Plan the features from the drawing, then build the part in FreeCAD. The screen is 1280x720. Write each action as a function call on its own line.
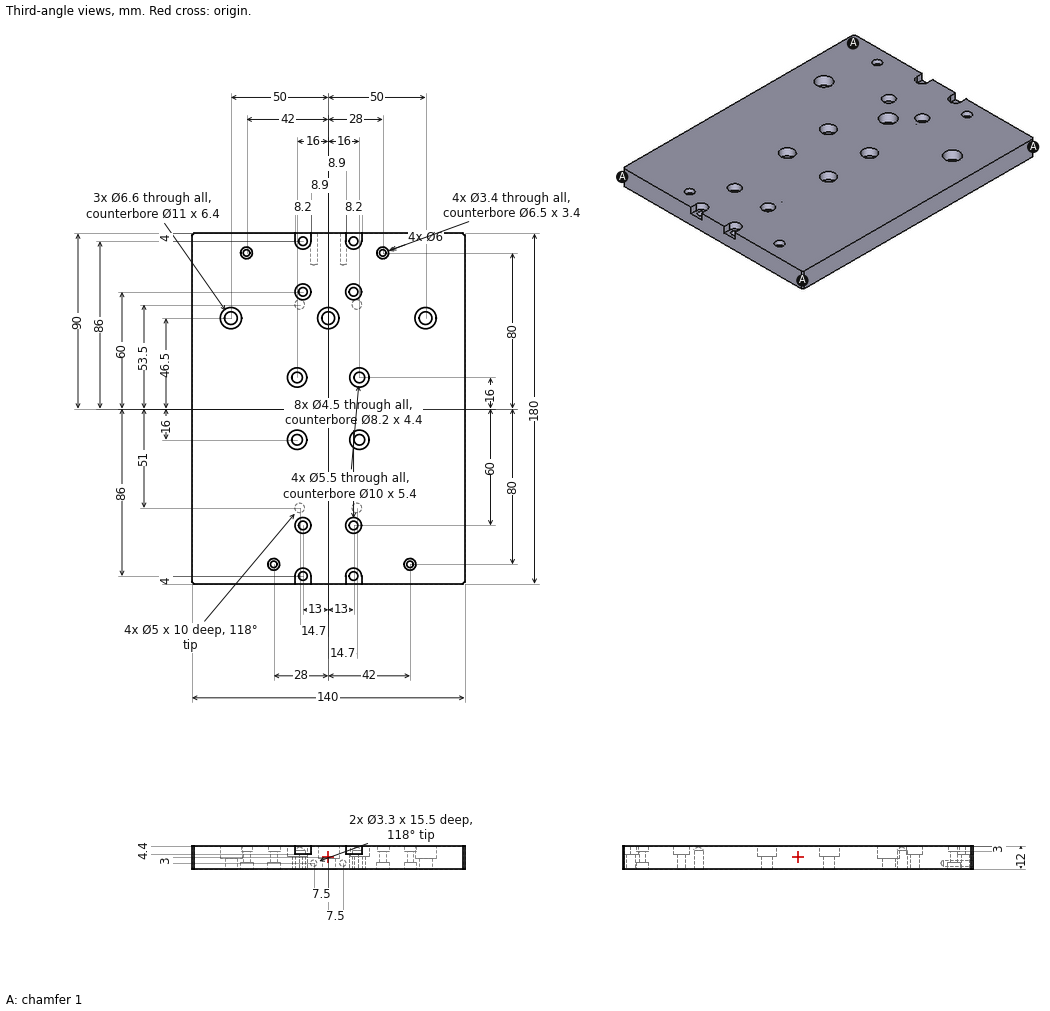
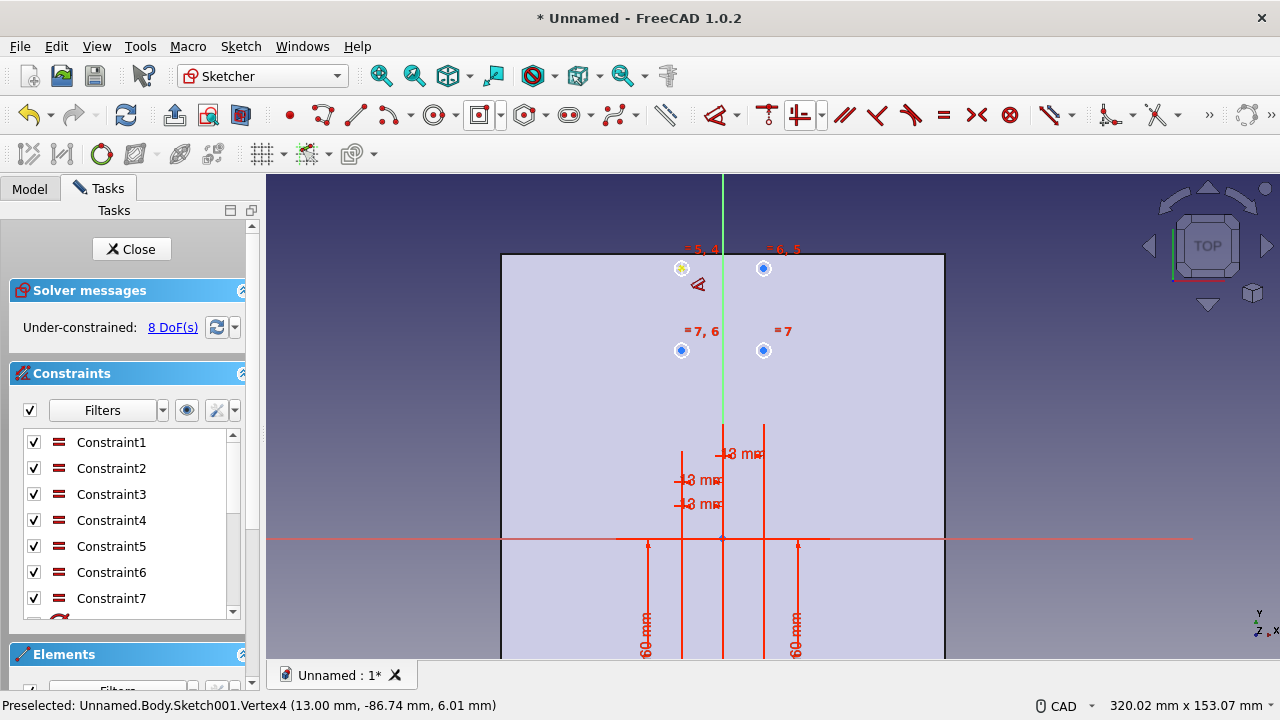
click(682, 269)
click(702, 235)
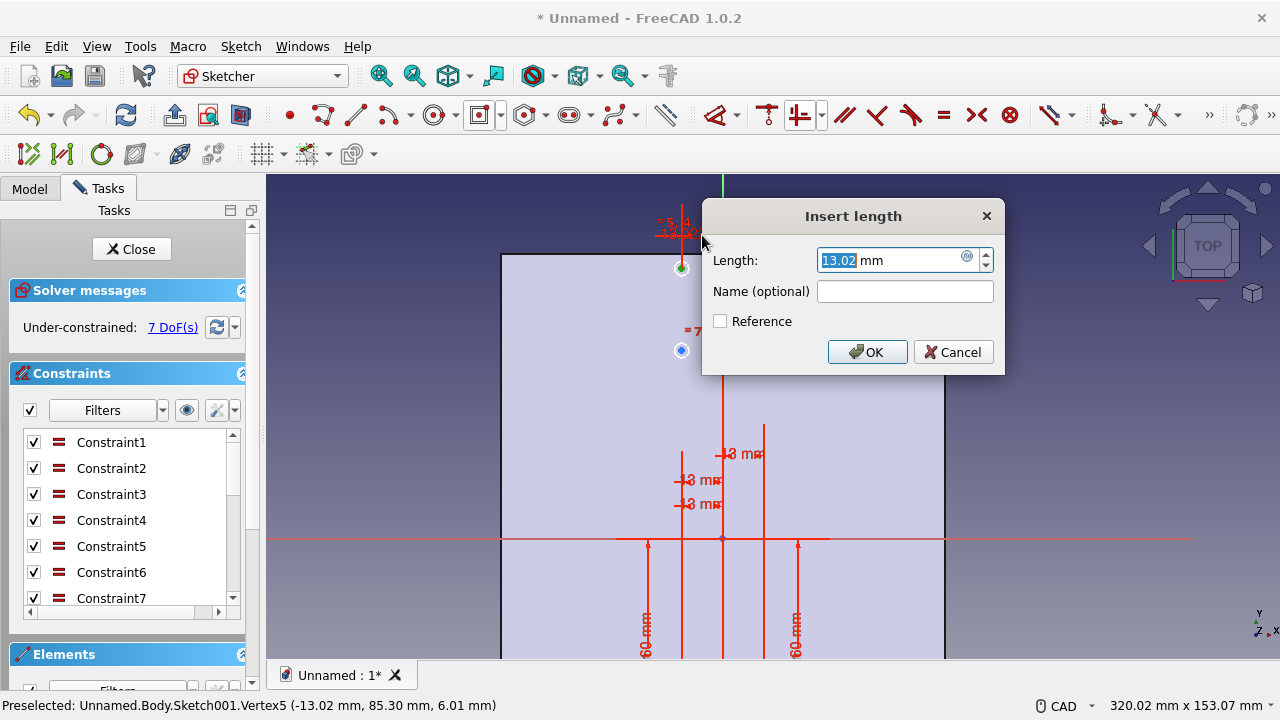
text(13)
key(Return)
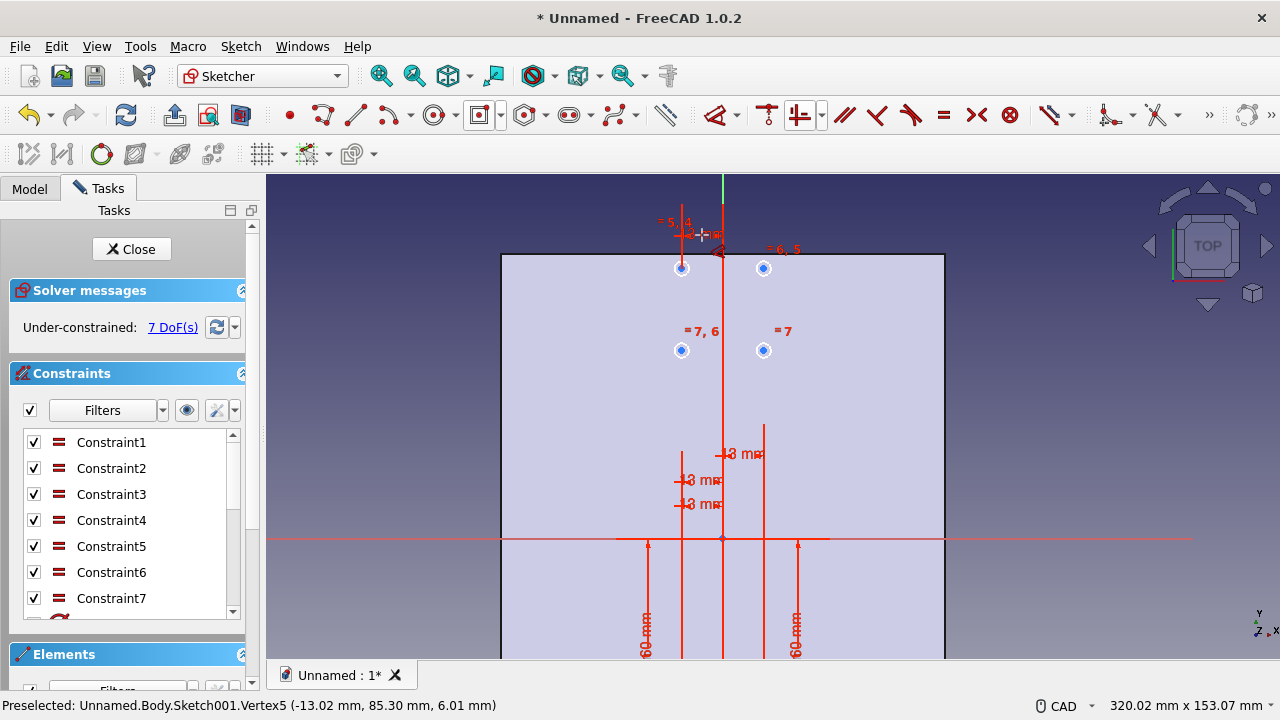
click(682, 269)
click(648, 404)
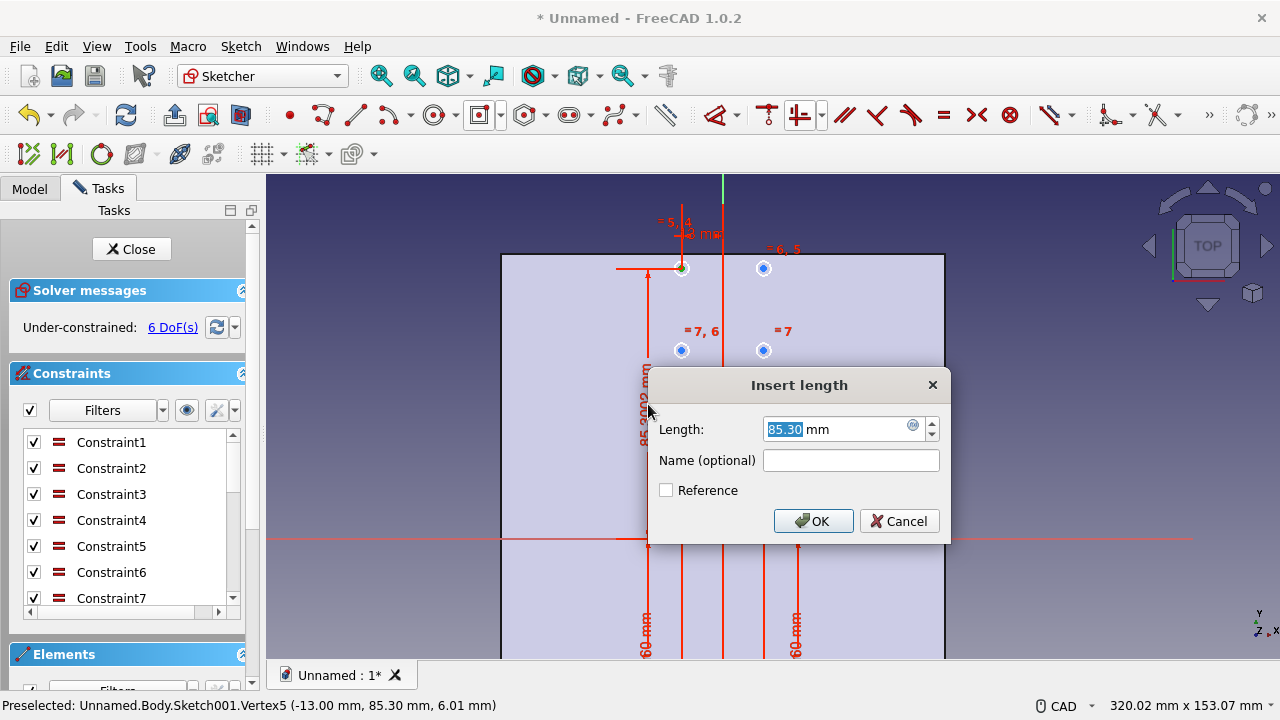
text(86)
key(Return)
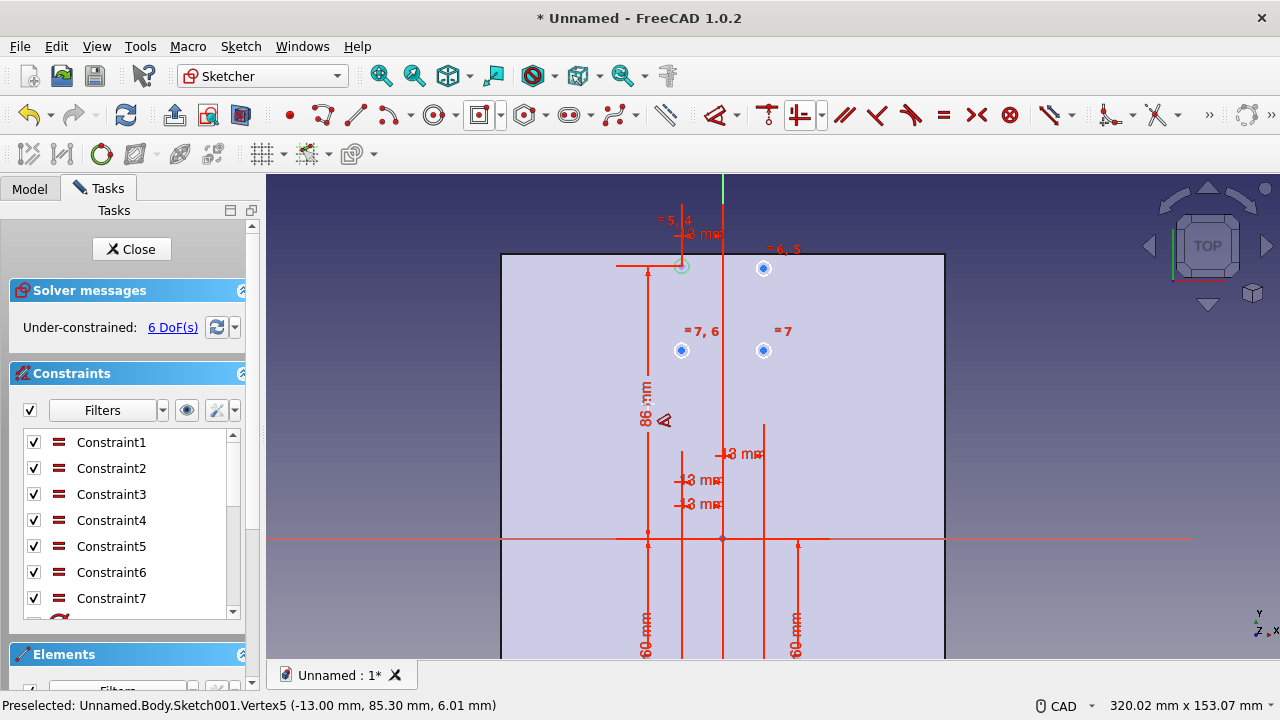
click(764, 269)
click(743, 573)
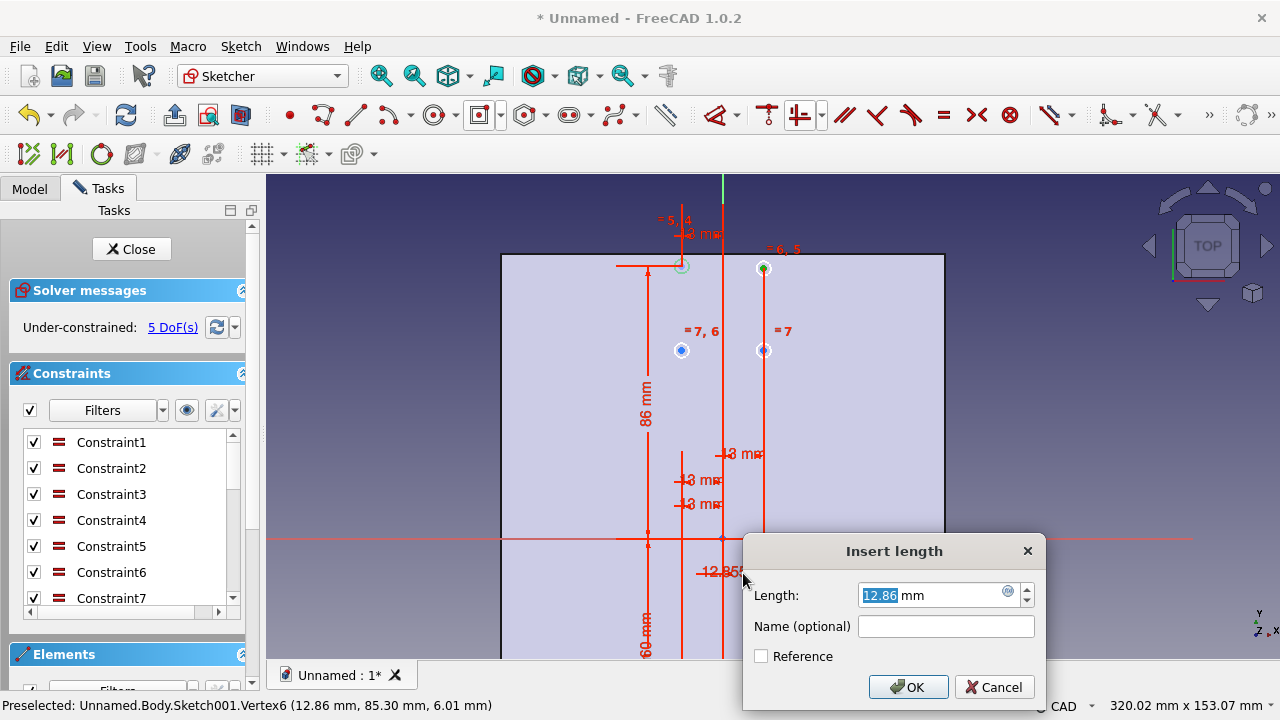
text(13)
key(Return)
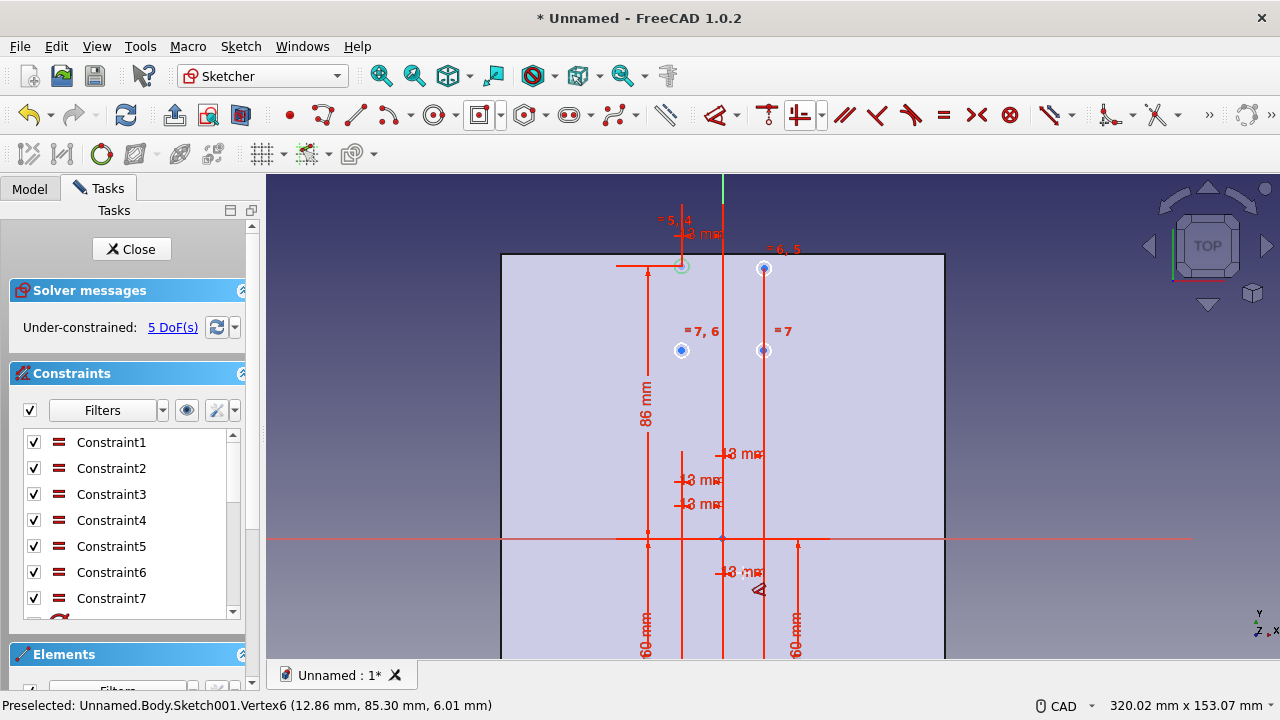
click(764, 269)
click(798, 404)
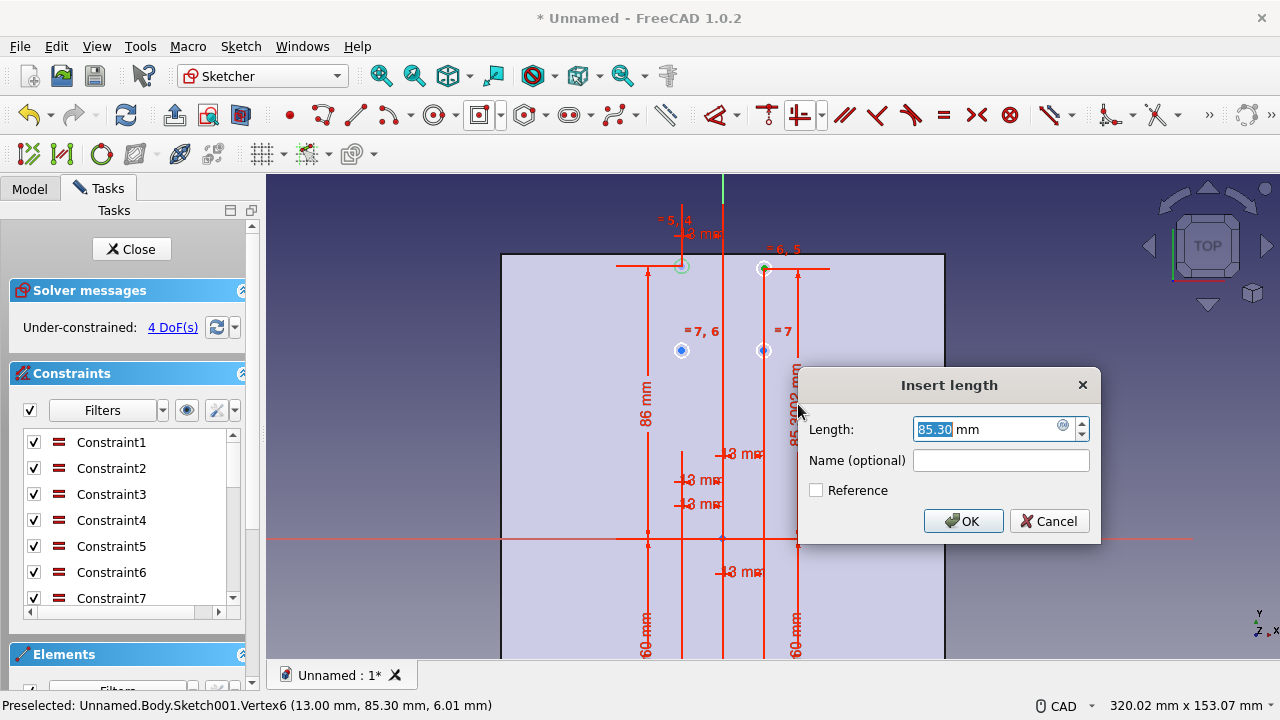
text(86)
key(Return)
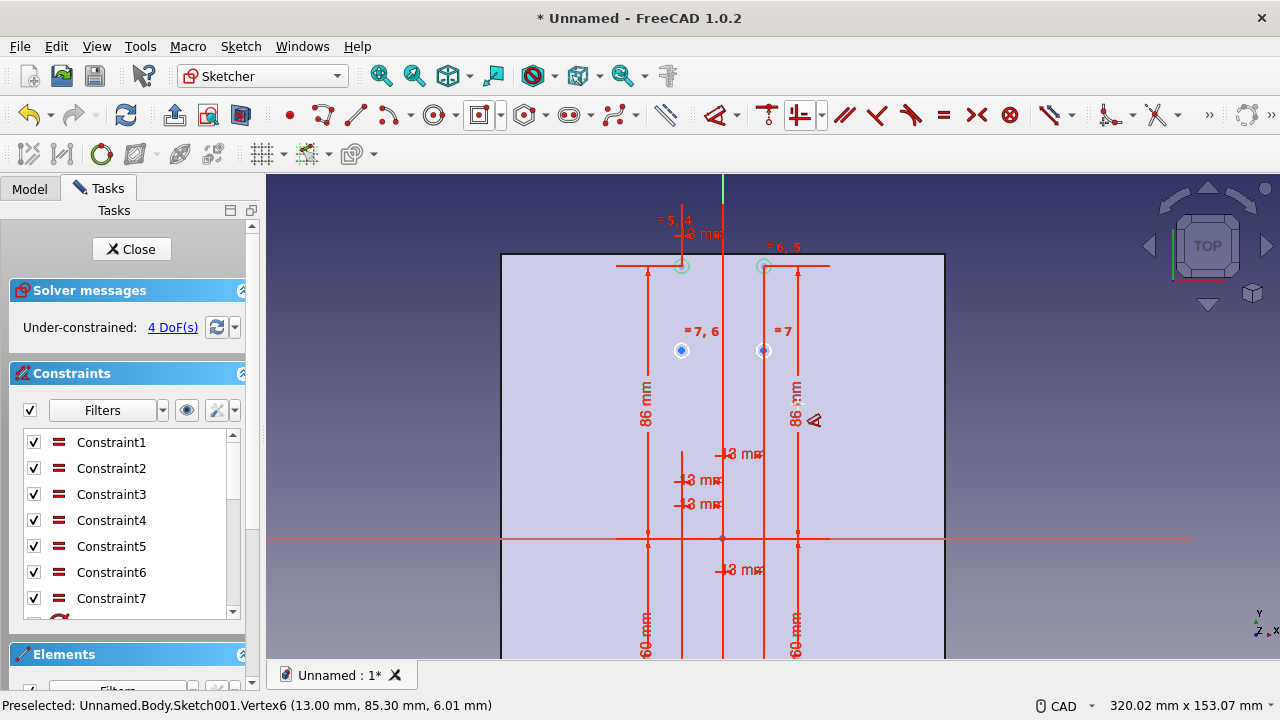
click(682, 351)
click(702, 317)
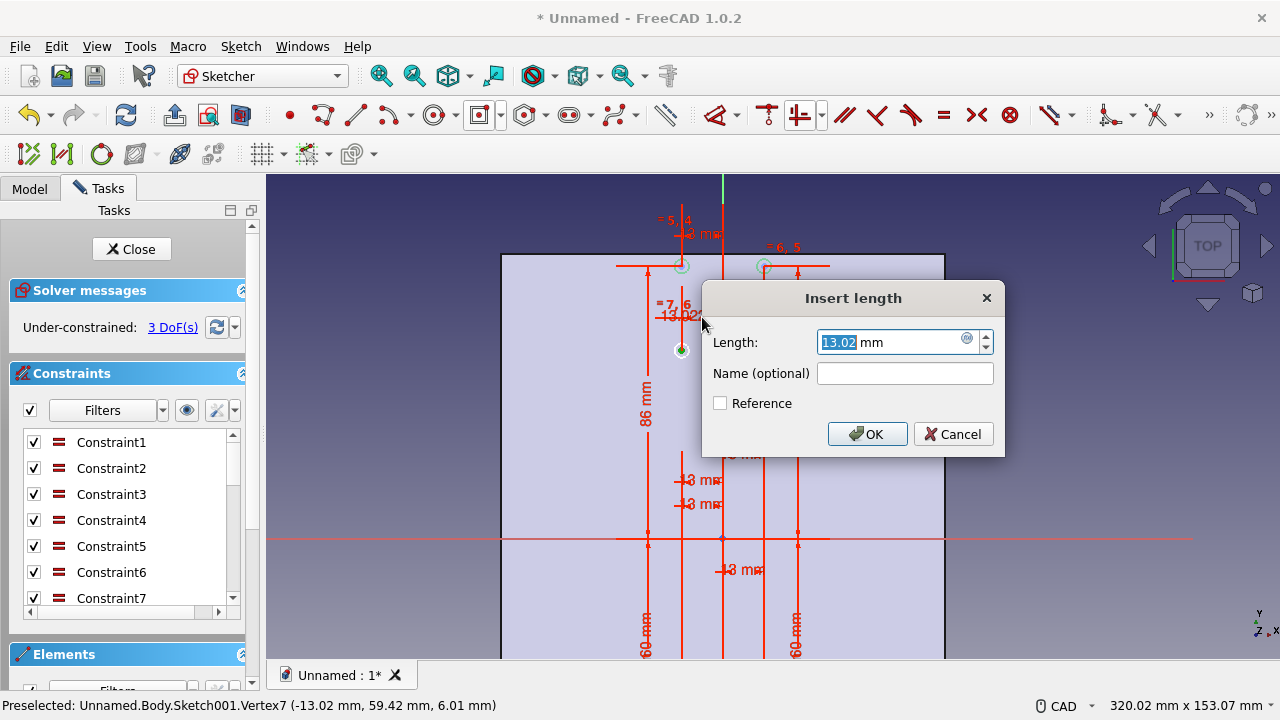
text(13)
key(Return)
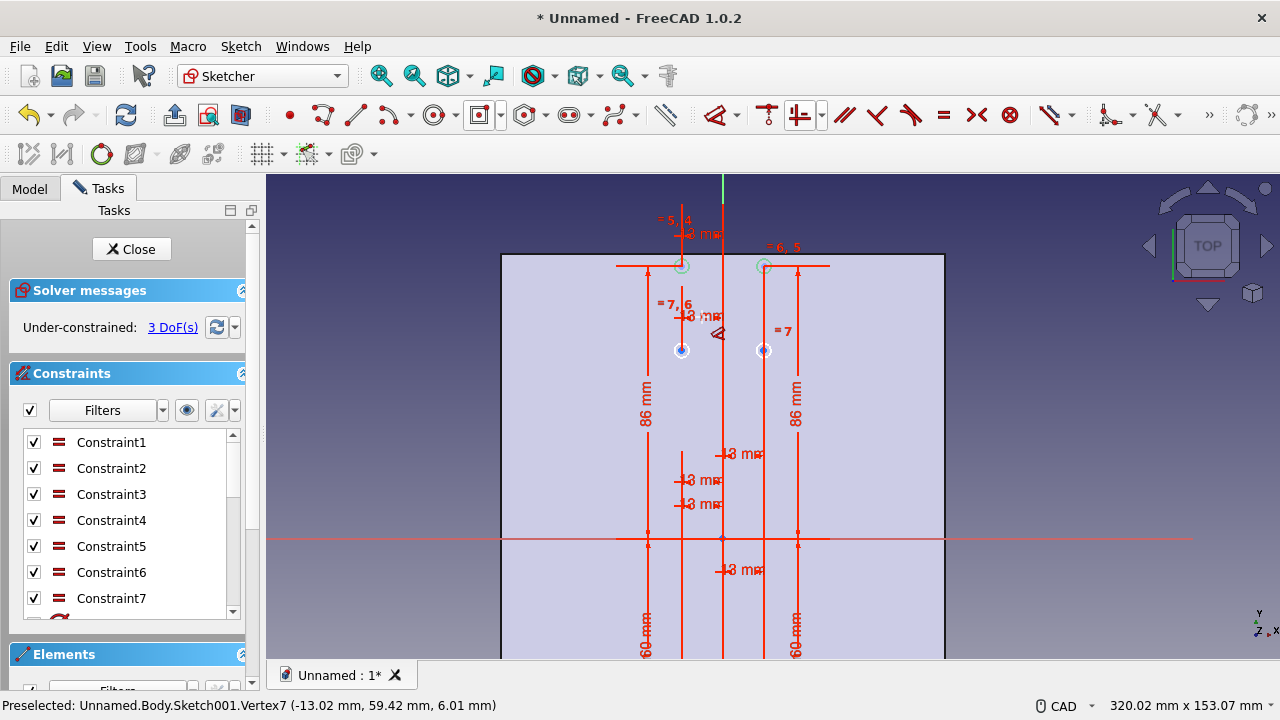
click(682, 351)
click(648, 445)